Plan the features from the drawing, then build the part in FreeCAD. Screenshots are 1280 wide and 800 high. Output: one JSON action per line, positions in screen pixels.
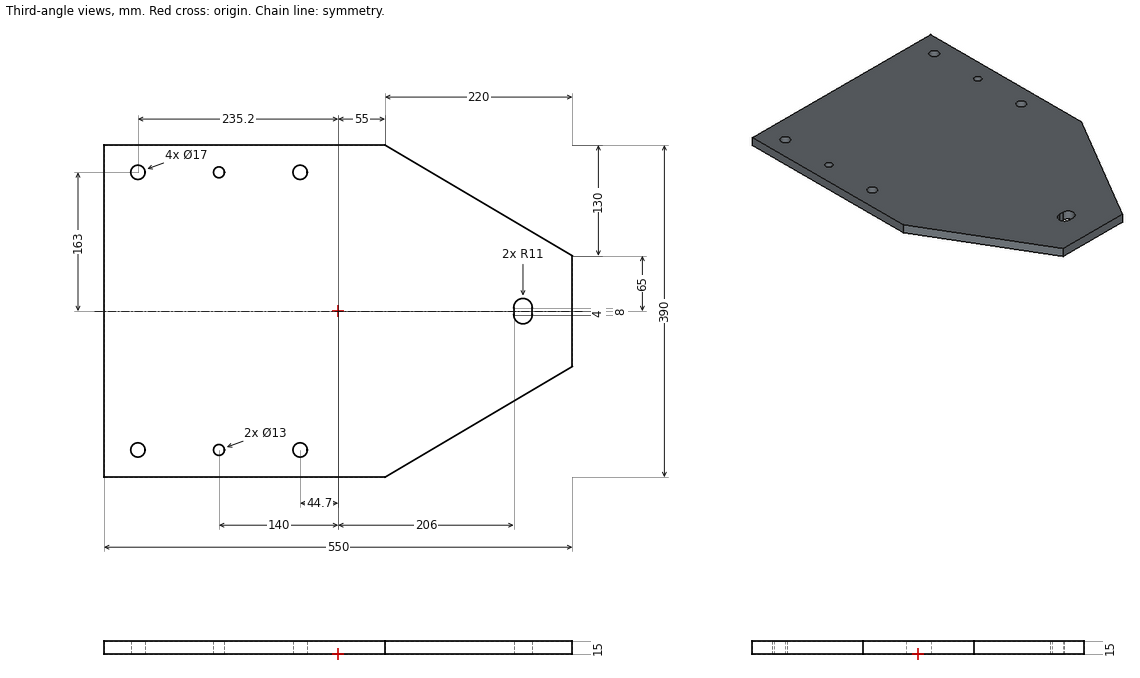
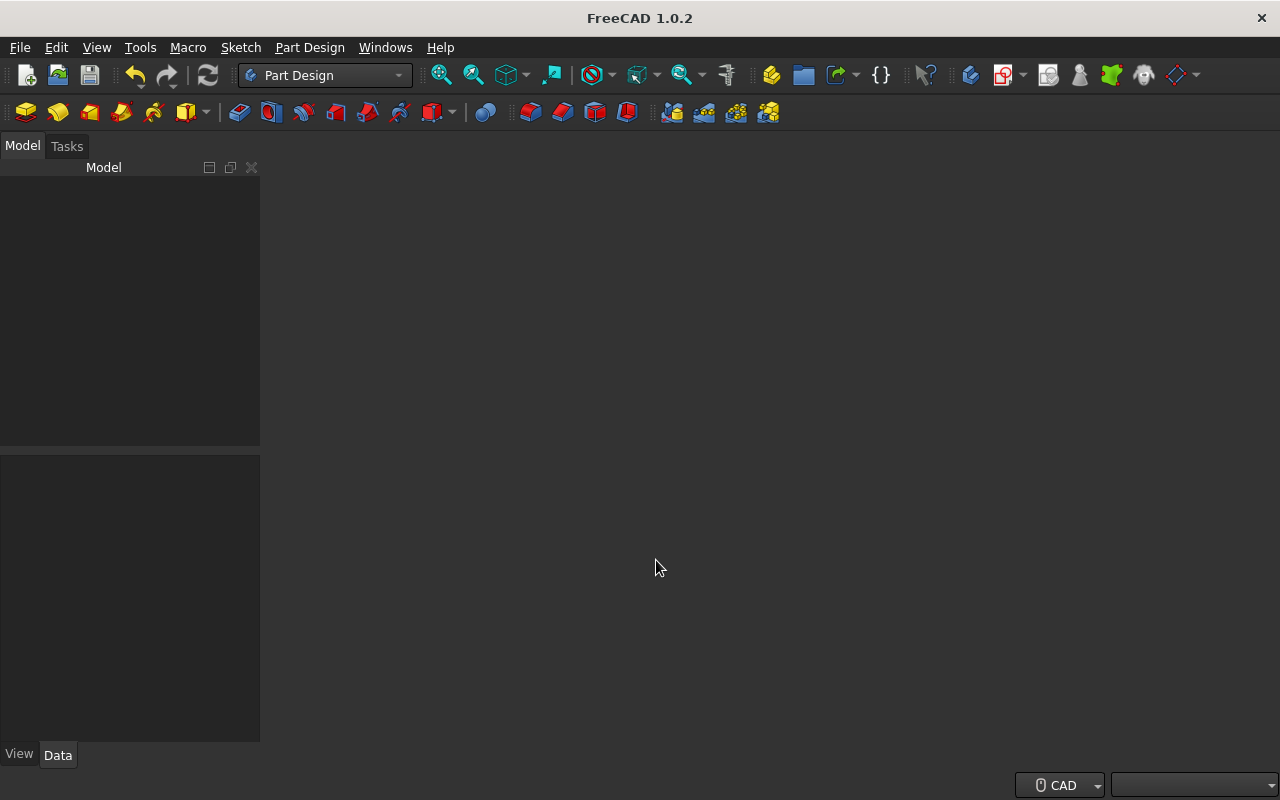
{"action": "left_click", "coordinate": [26, 76]}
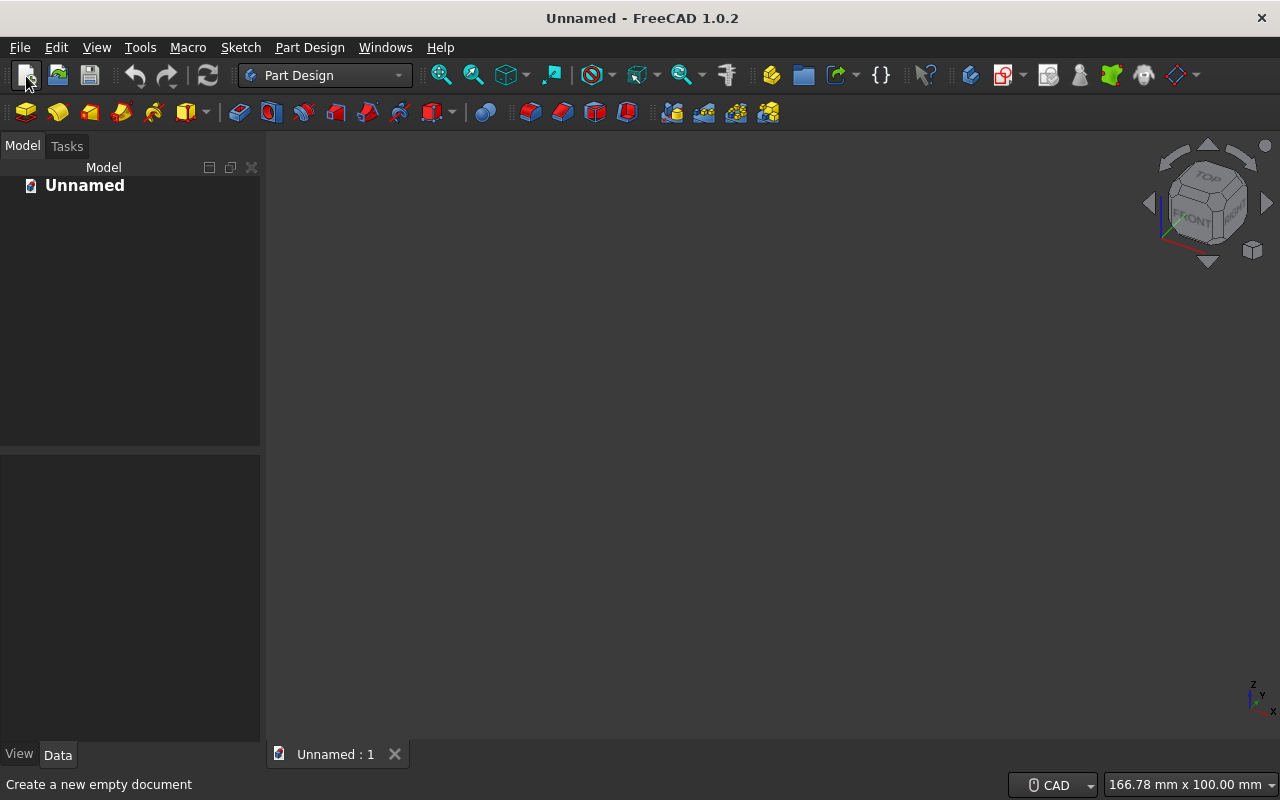
{"action": "left_click", "coordinate": [1004, 76]}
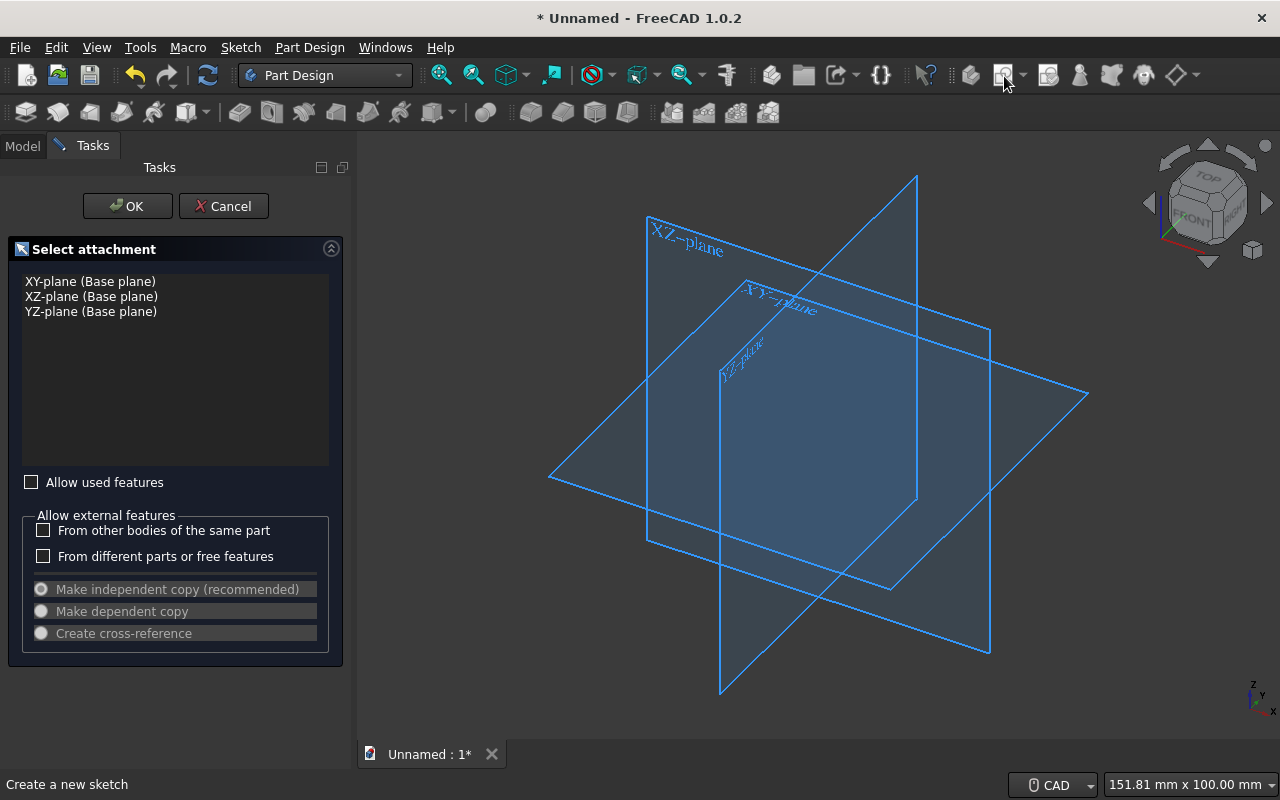
{"action": "left_click", "coordinate": [82, 282]}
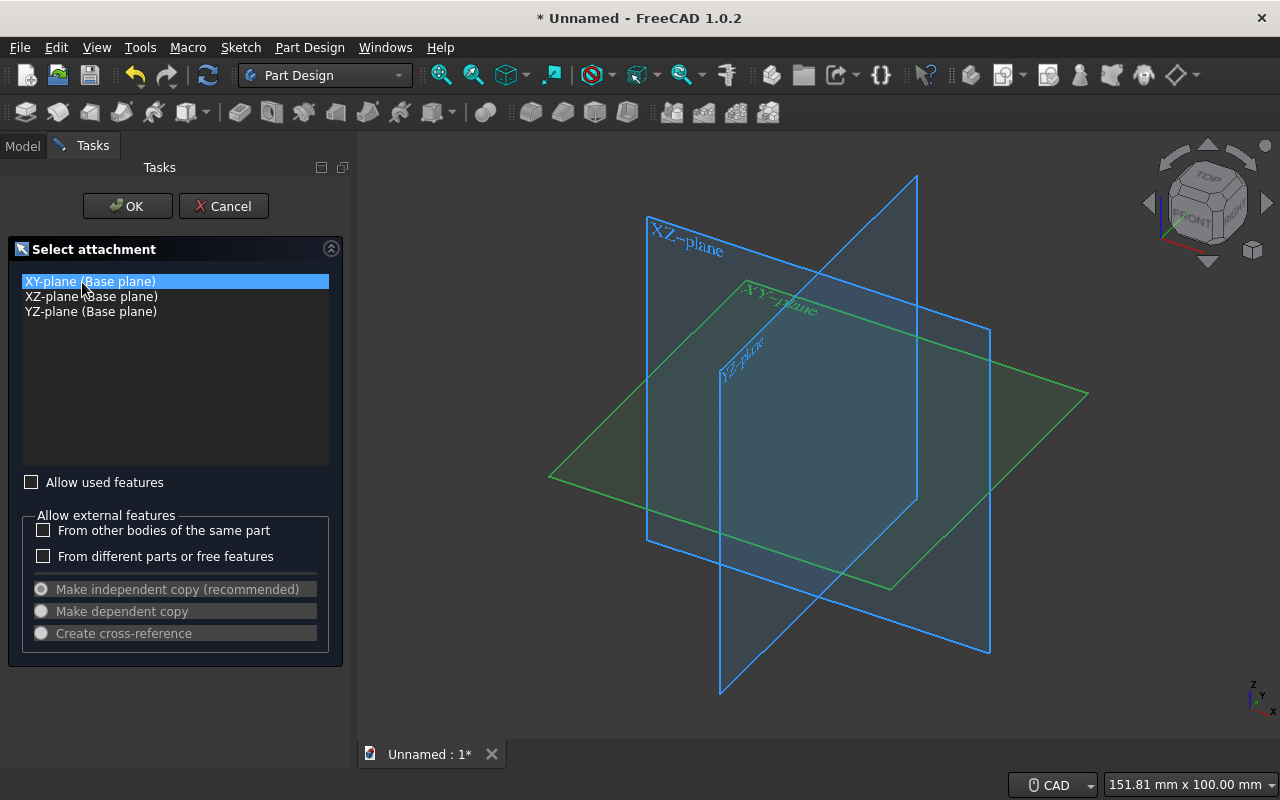
{"action": "left_click", "coordinate": [128, 206]}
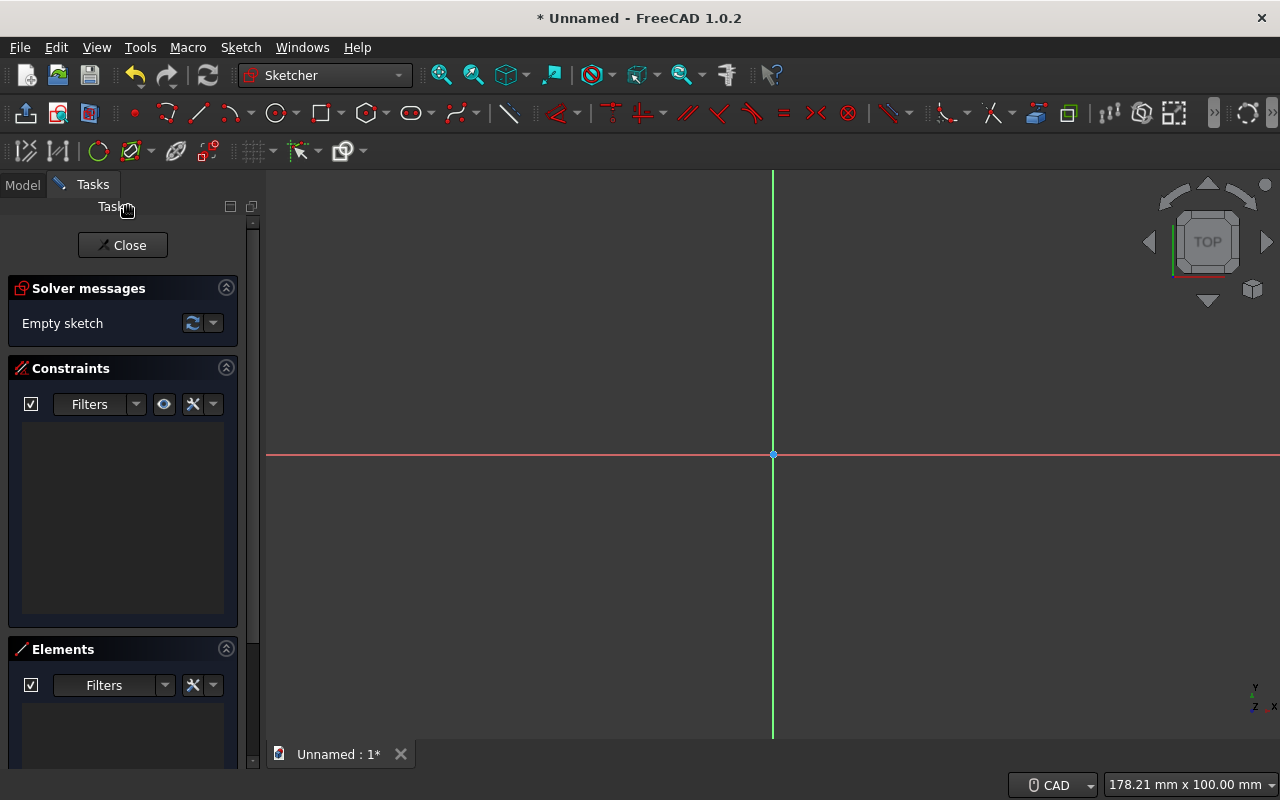
{"action": "scroll", "coordinate": [691, 454], "scroll_direction": "down", "scroll_amount": 9}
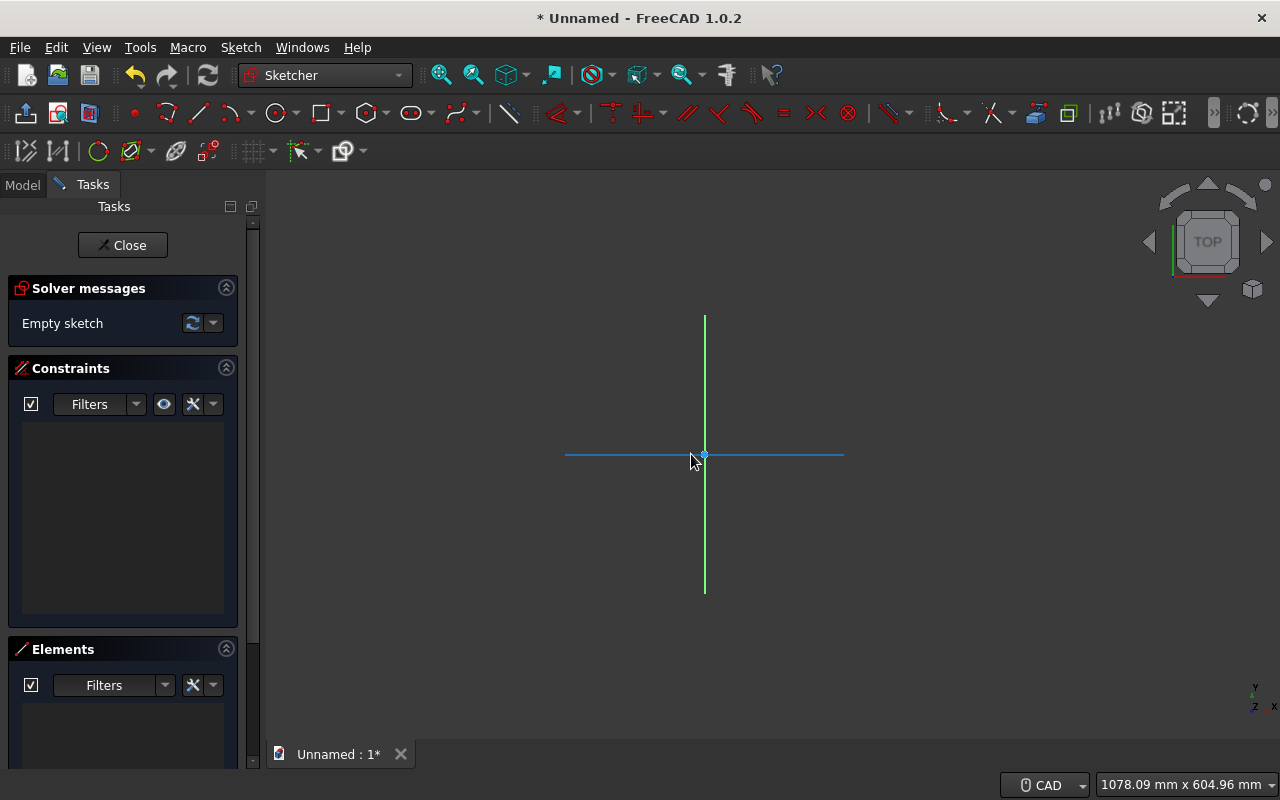
{"action": "left_click", "coordinate": [344, 114]}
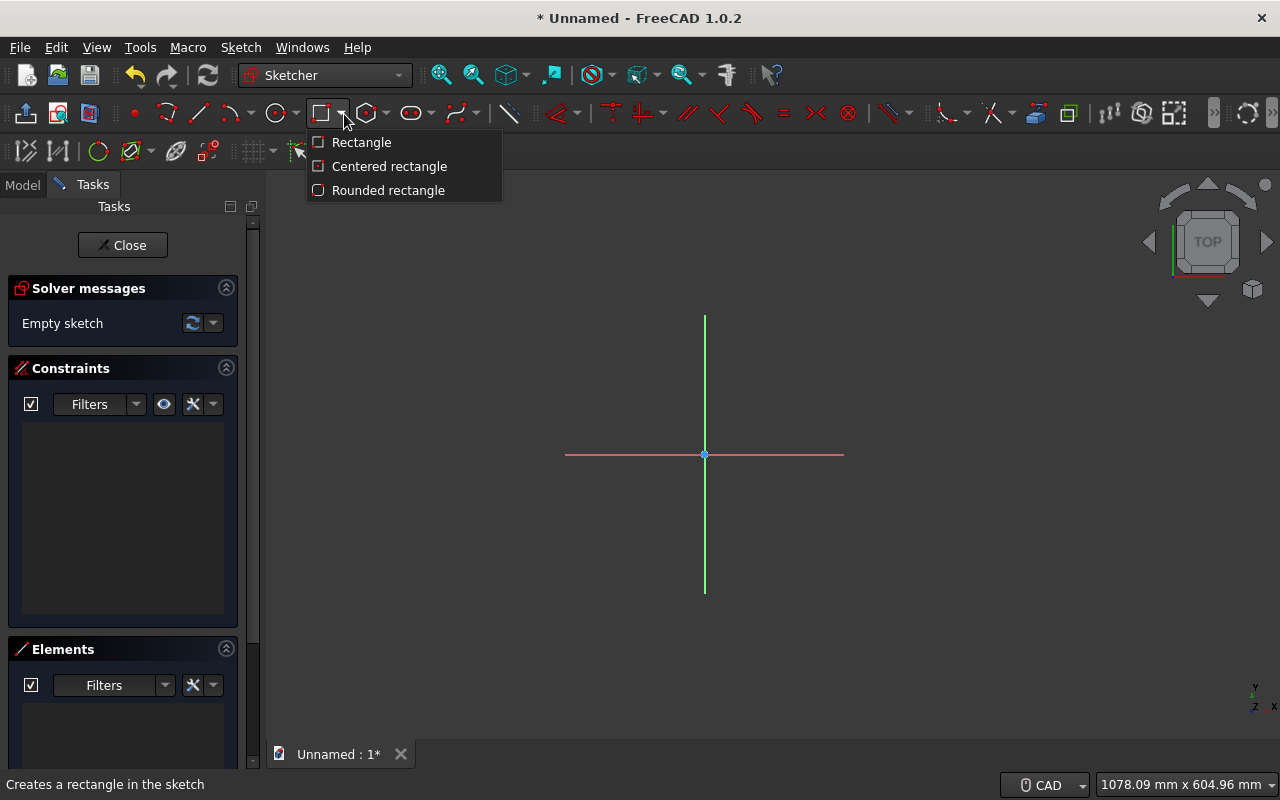
{"action": "left_click", "coordinate": [404, 166]}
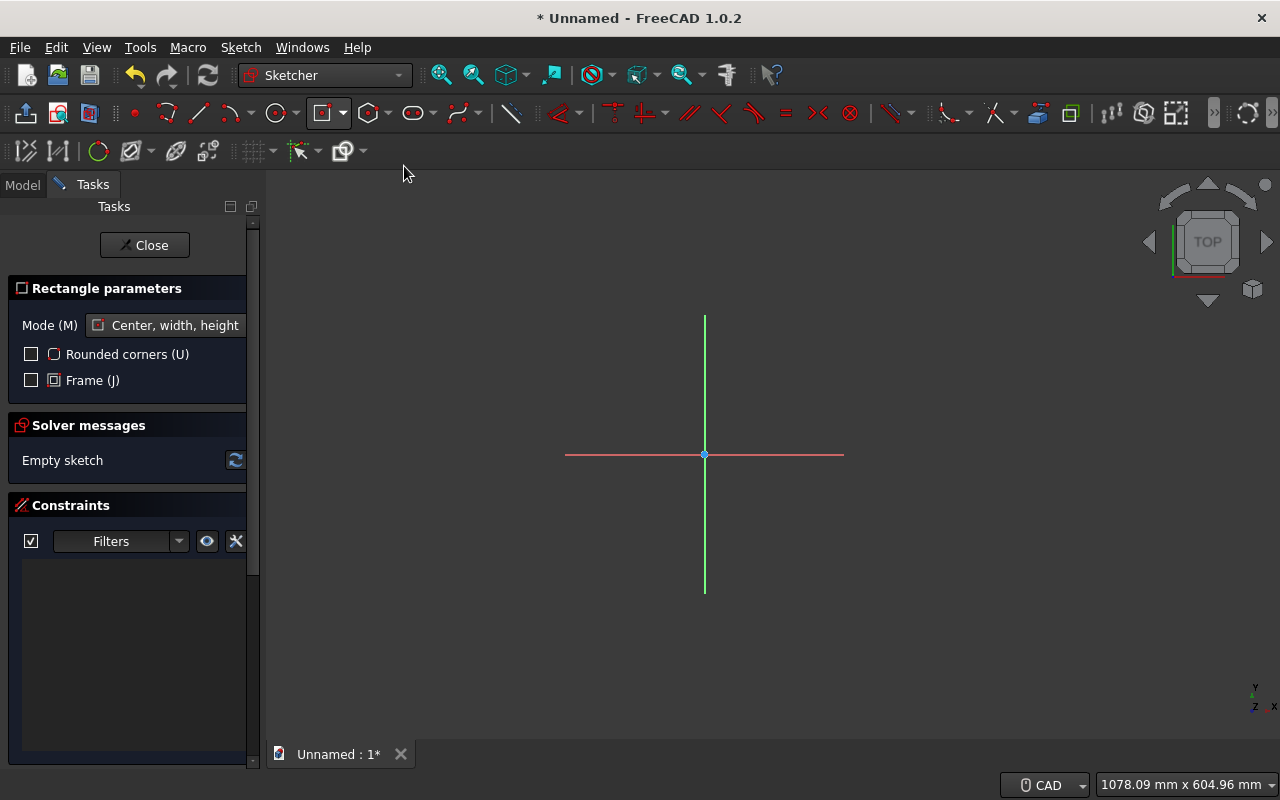
{"action": "left_click", "coordinate": [705, 454]}
{"action": "left_click", "coordinate": [964, 271]}
{"action": "key", "text": "Escape"}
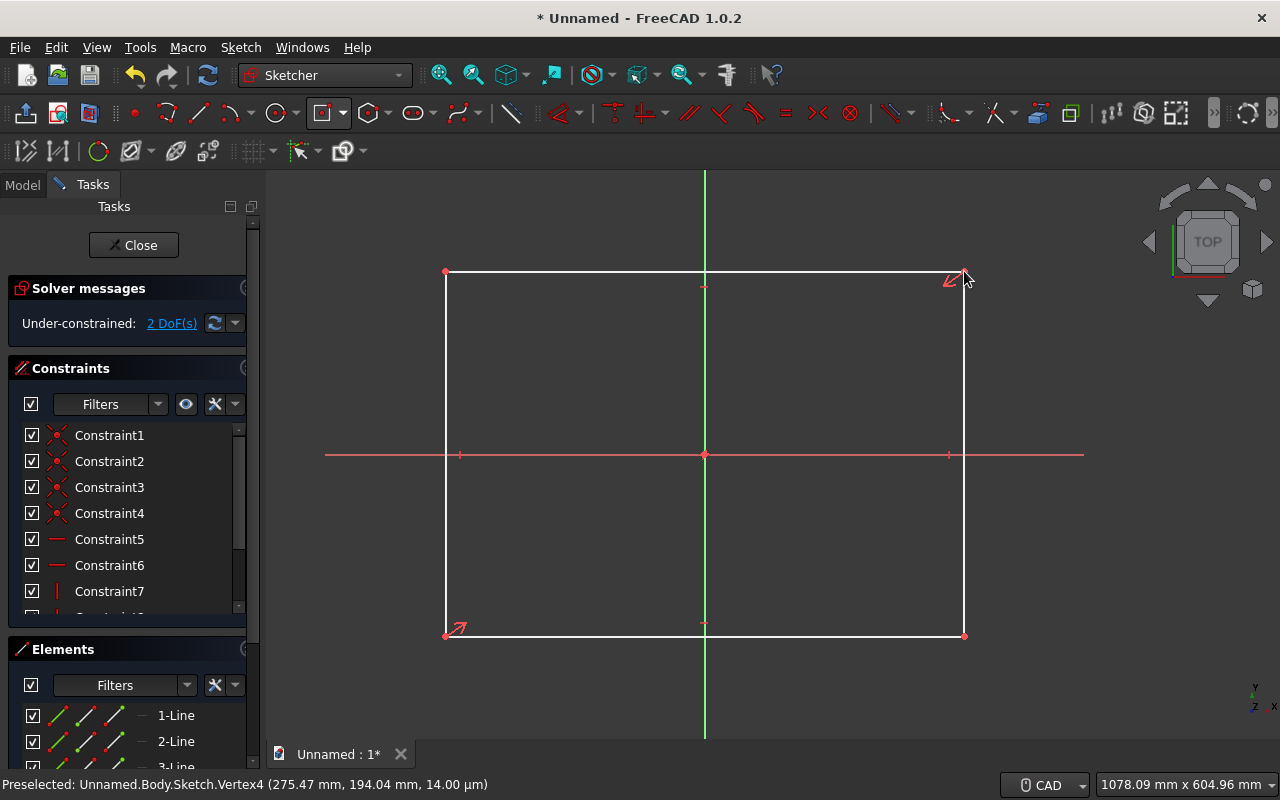
{"action": "left_click", "coordinate": [558, 114]}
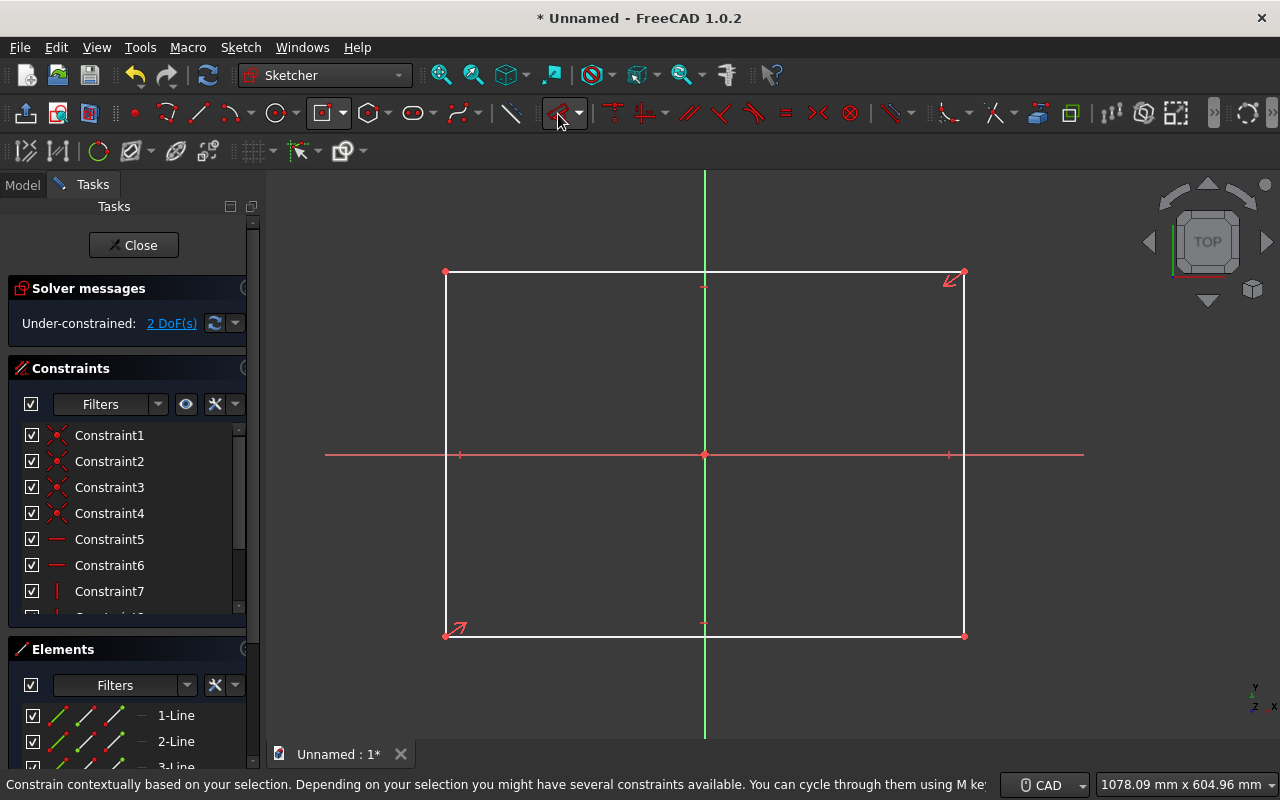
{"action": "left_click", "coordinate": [601, 637]}
{"action": "left_click", "coordinate": [586, 671]}